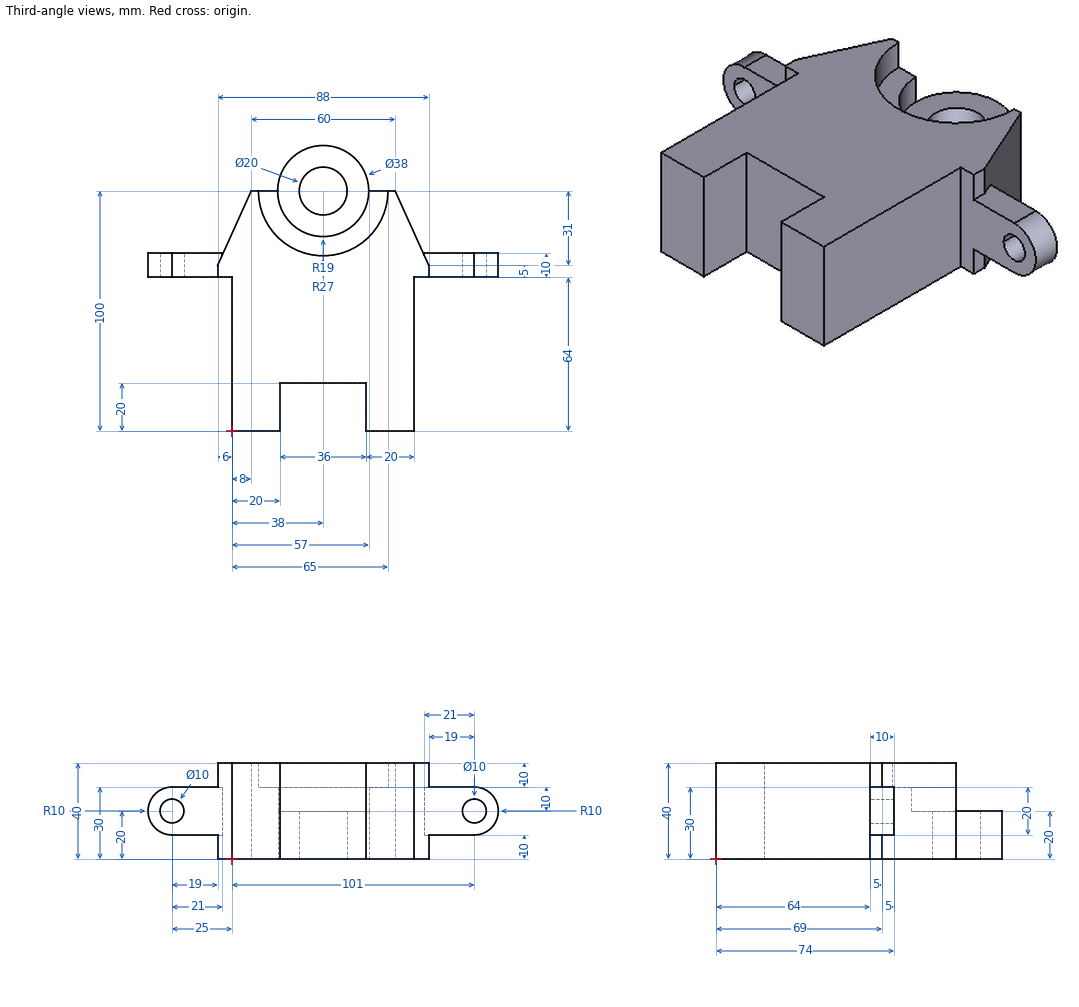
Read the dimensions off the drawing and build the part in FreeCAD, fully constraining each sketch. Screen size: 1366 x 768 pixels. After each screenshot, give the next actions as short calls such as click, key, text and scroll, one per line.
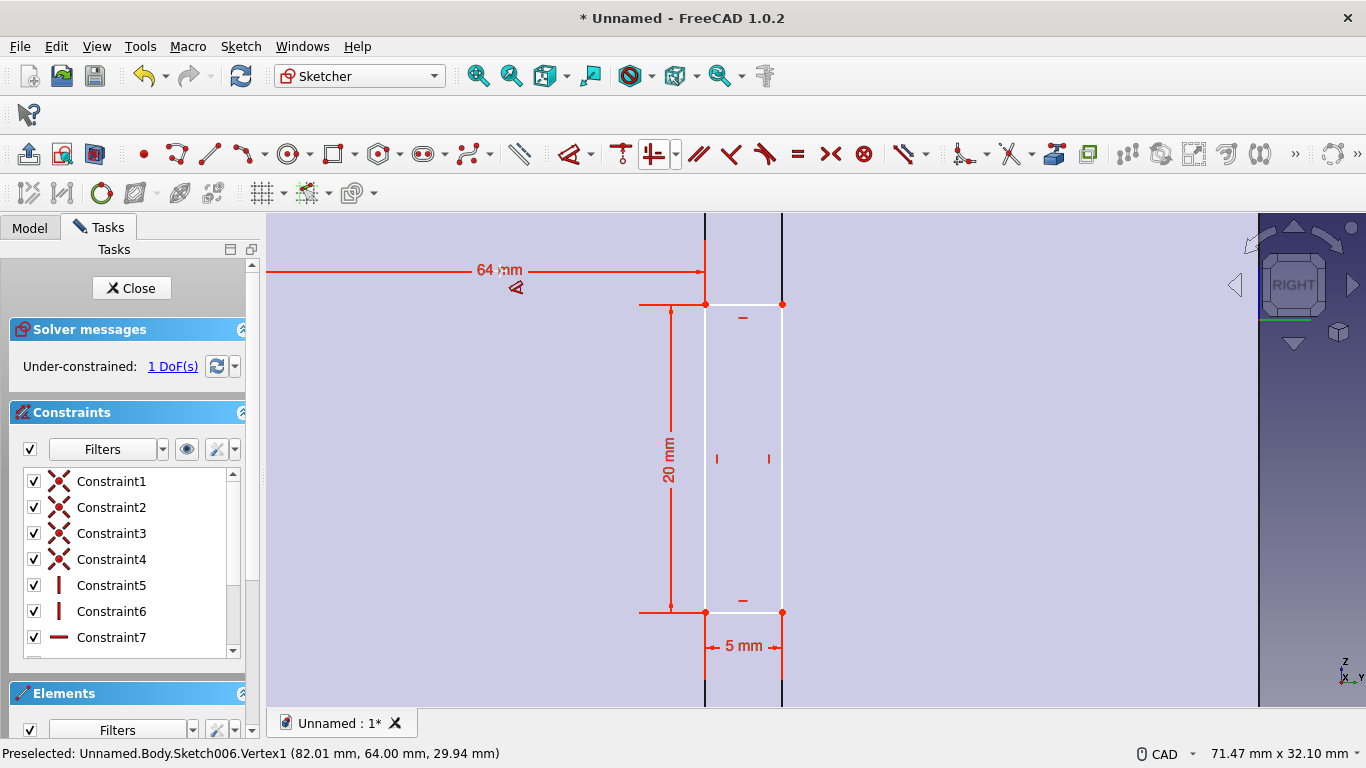
click(705, 305)
click(739, 492)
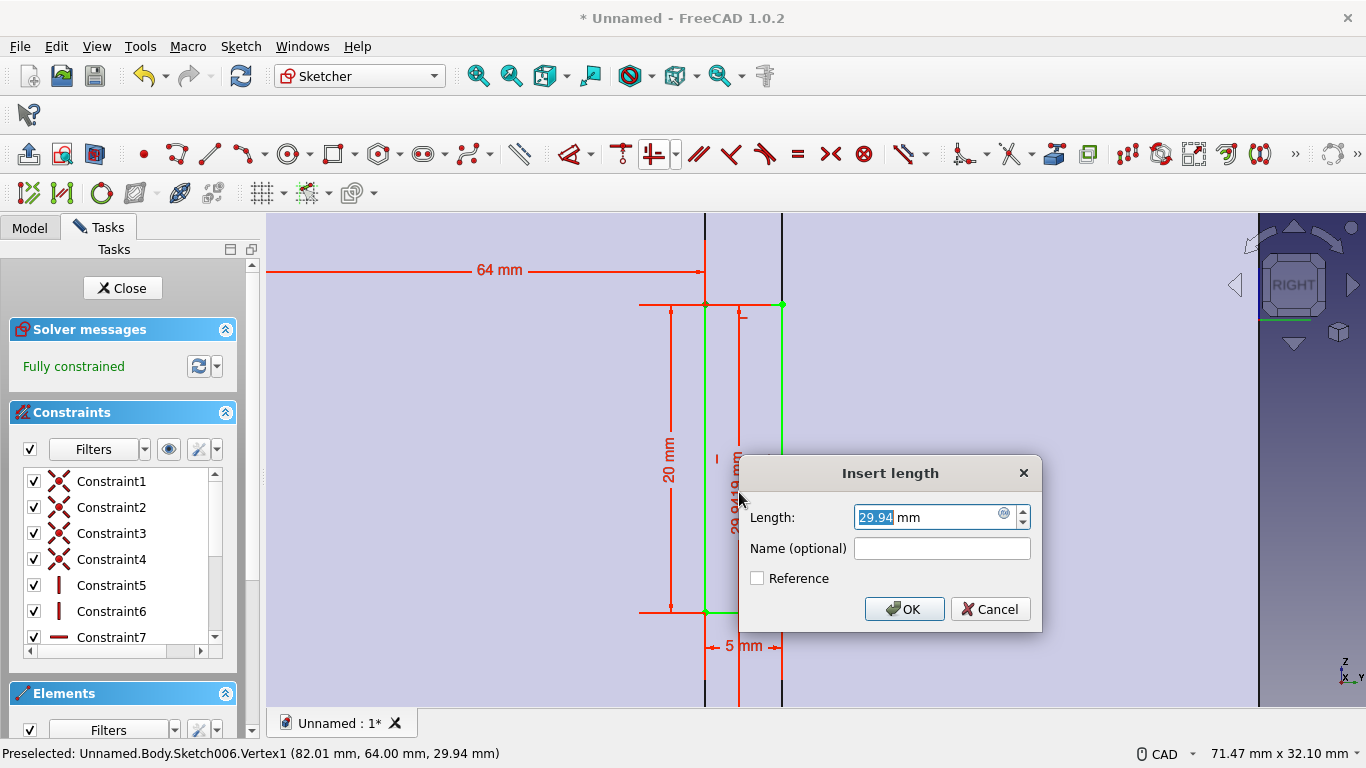
text(30)
key(Return)
key(Escape)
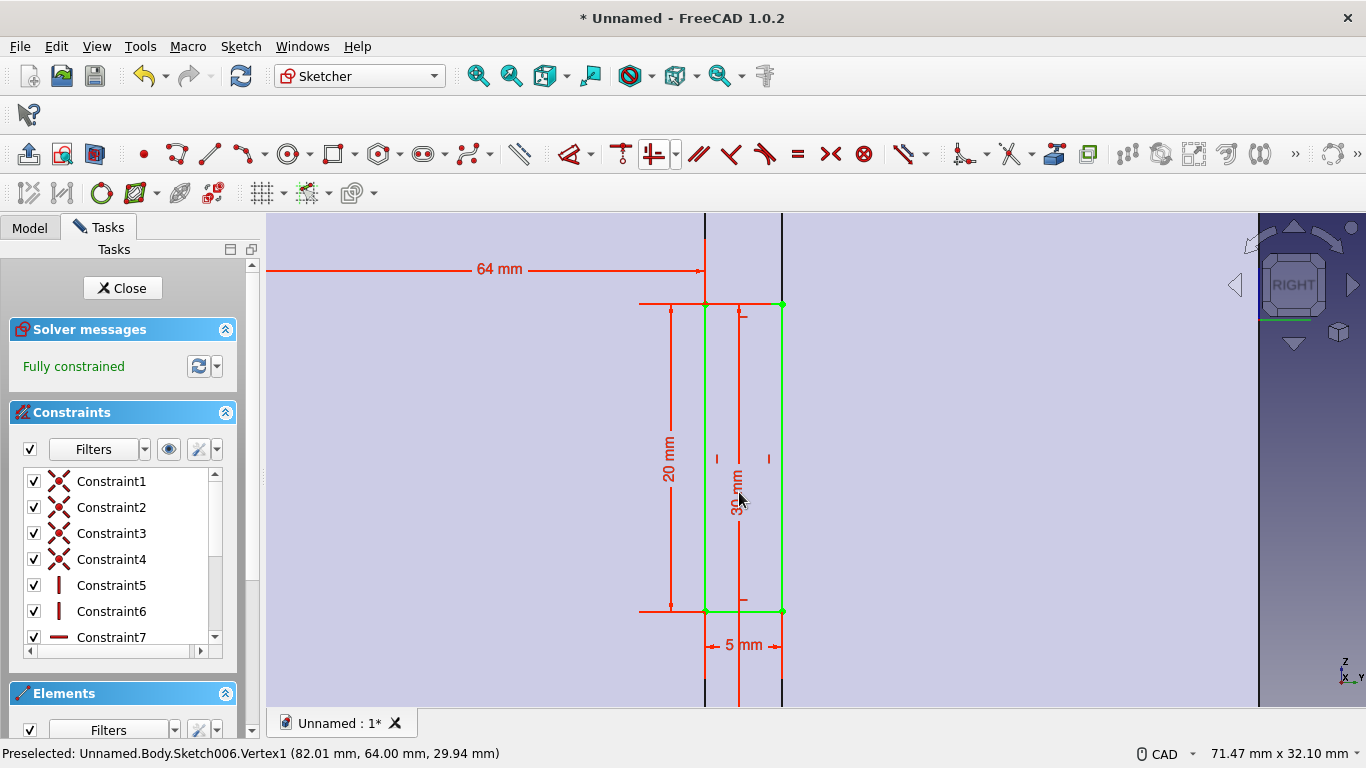
click(123, 288)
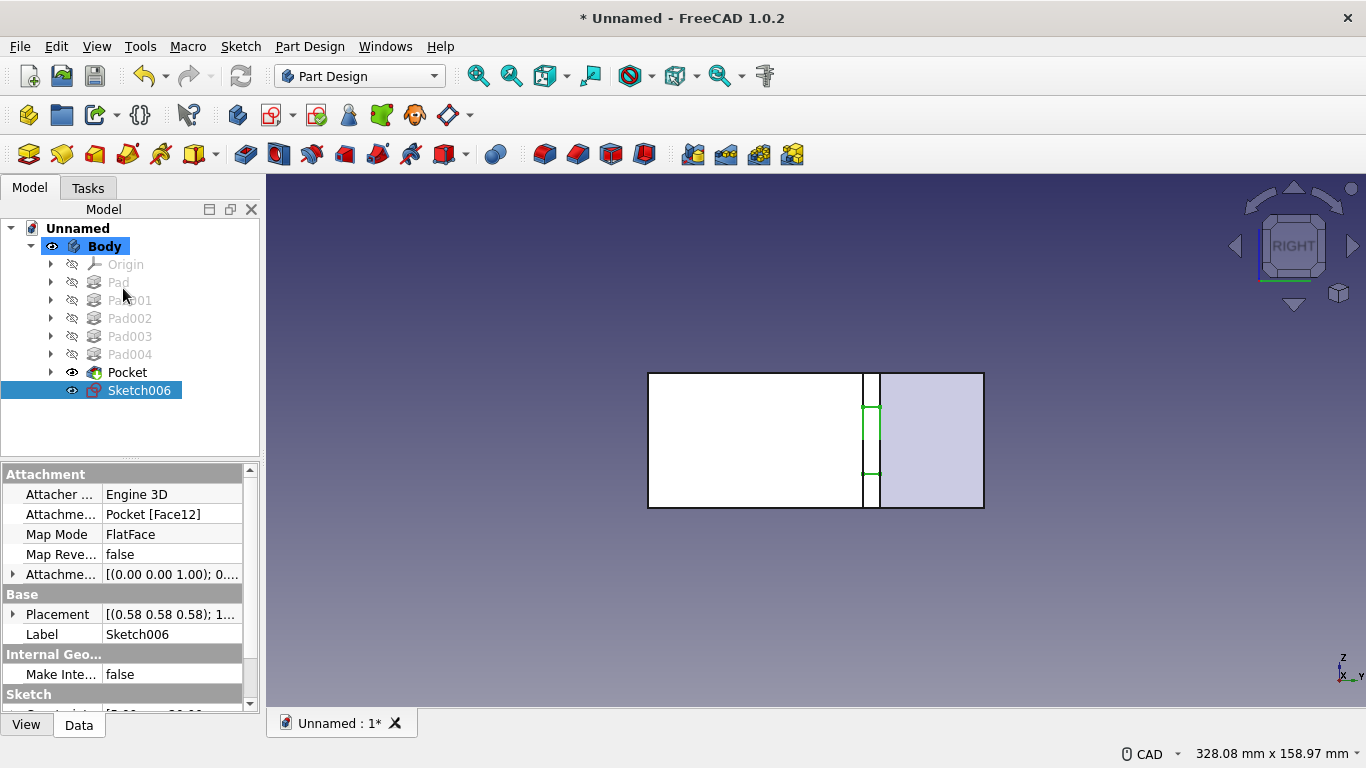
click(29, 154)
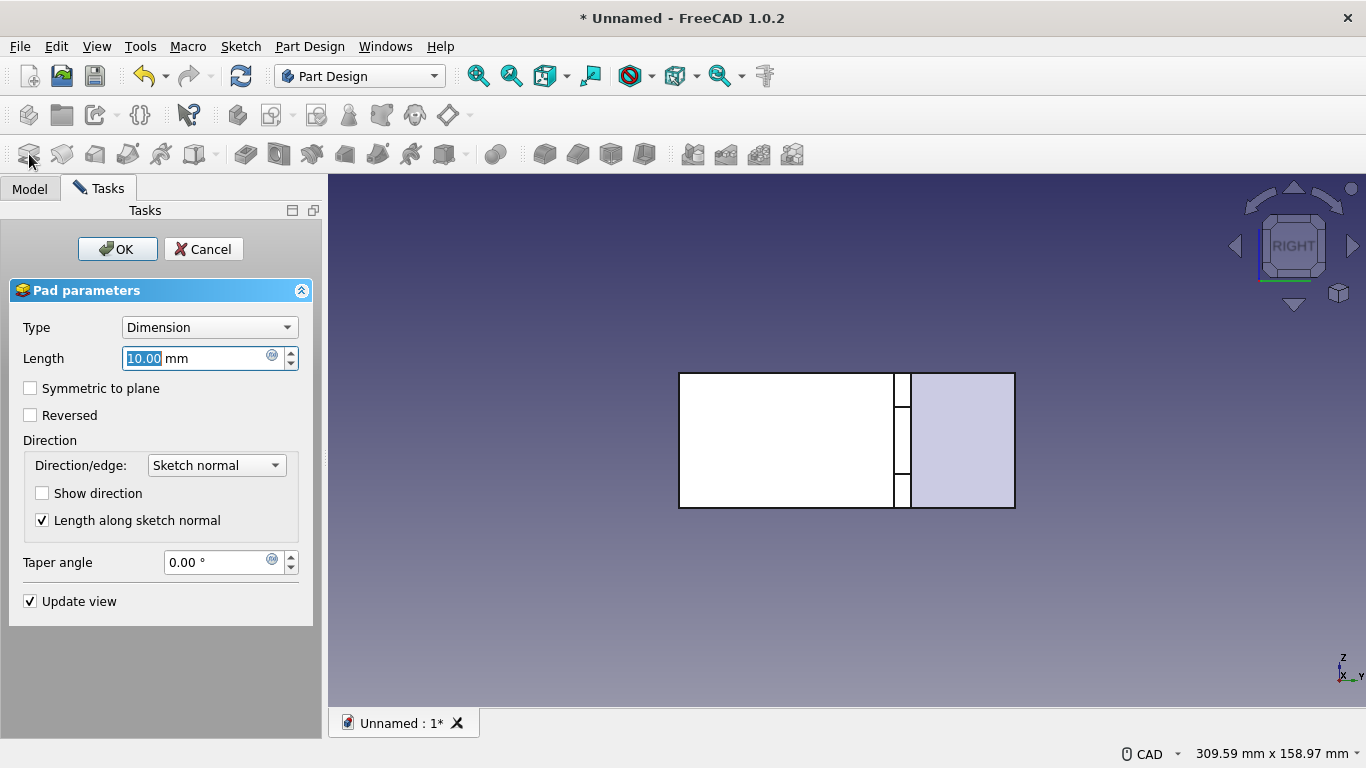
text(19)
key(Tab)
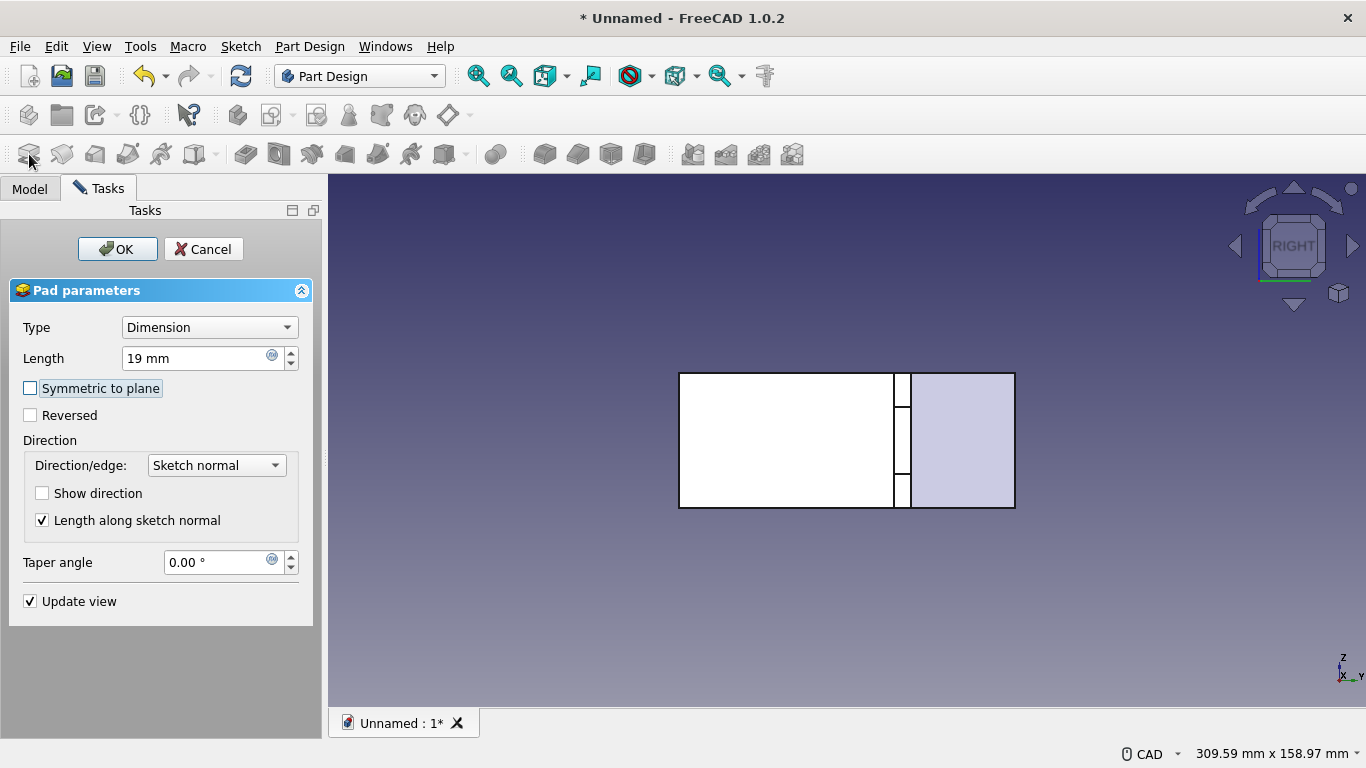
click(118, 249)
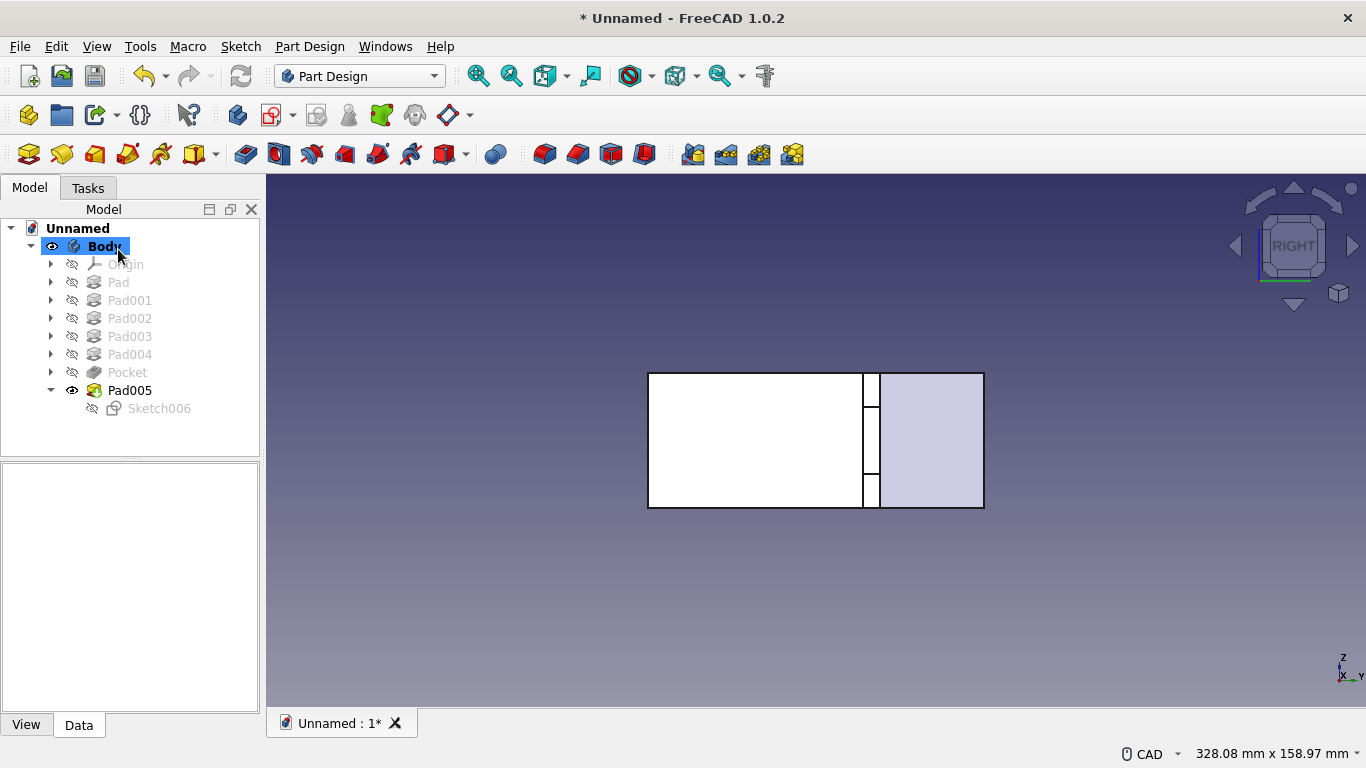
click(479, 76)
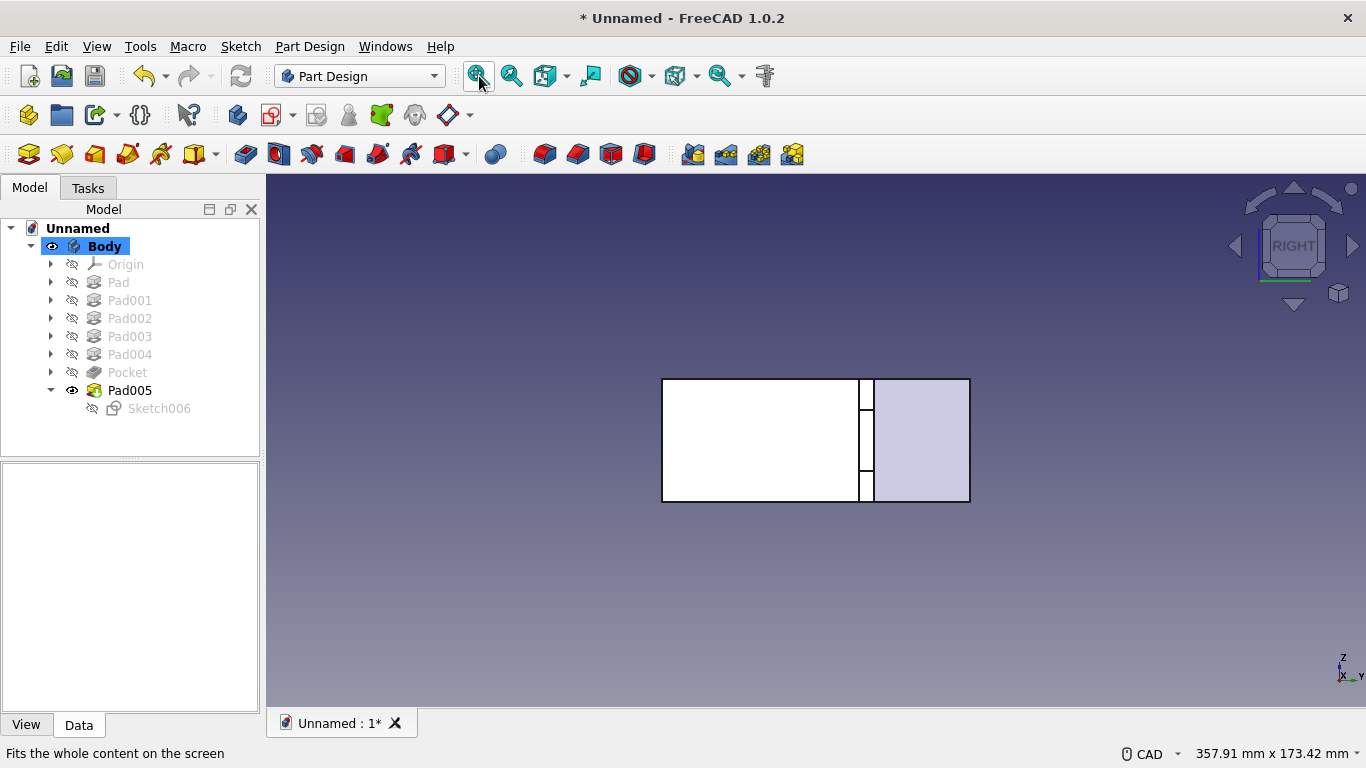
key(0)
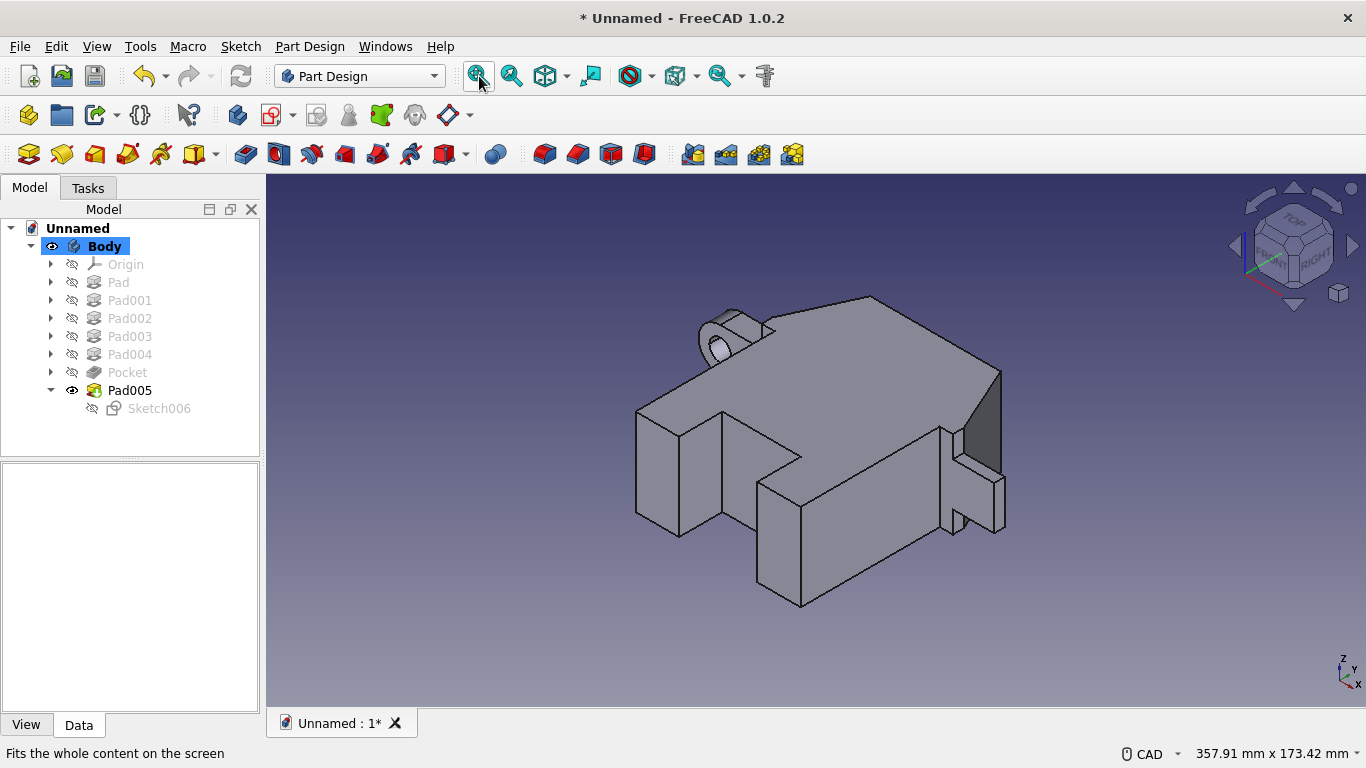
key(3)